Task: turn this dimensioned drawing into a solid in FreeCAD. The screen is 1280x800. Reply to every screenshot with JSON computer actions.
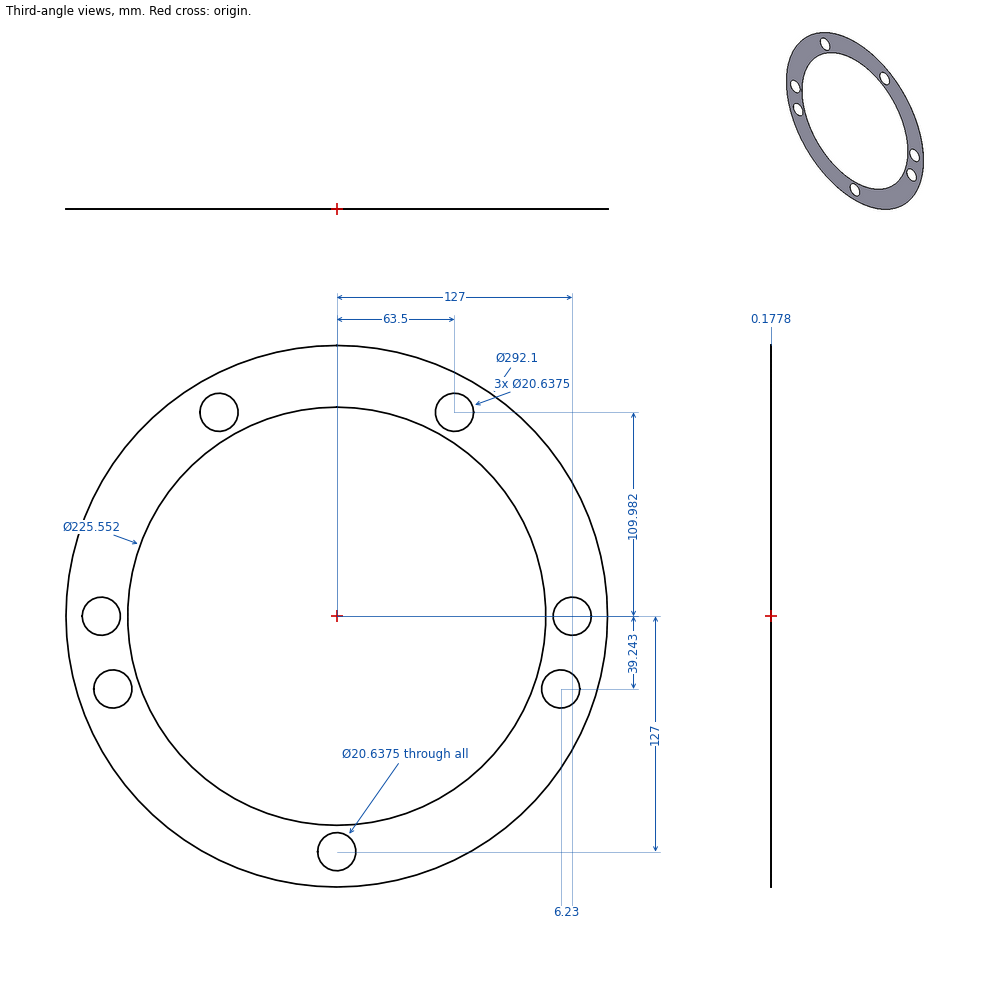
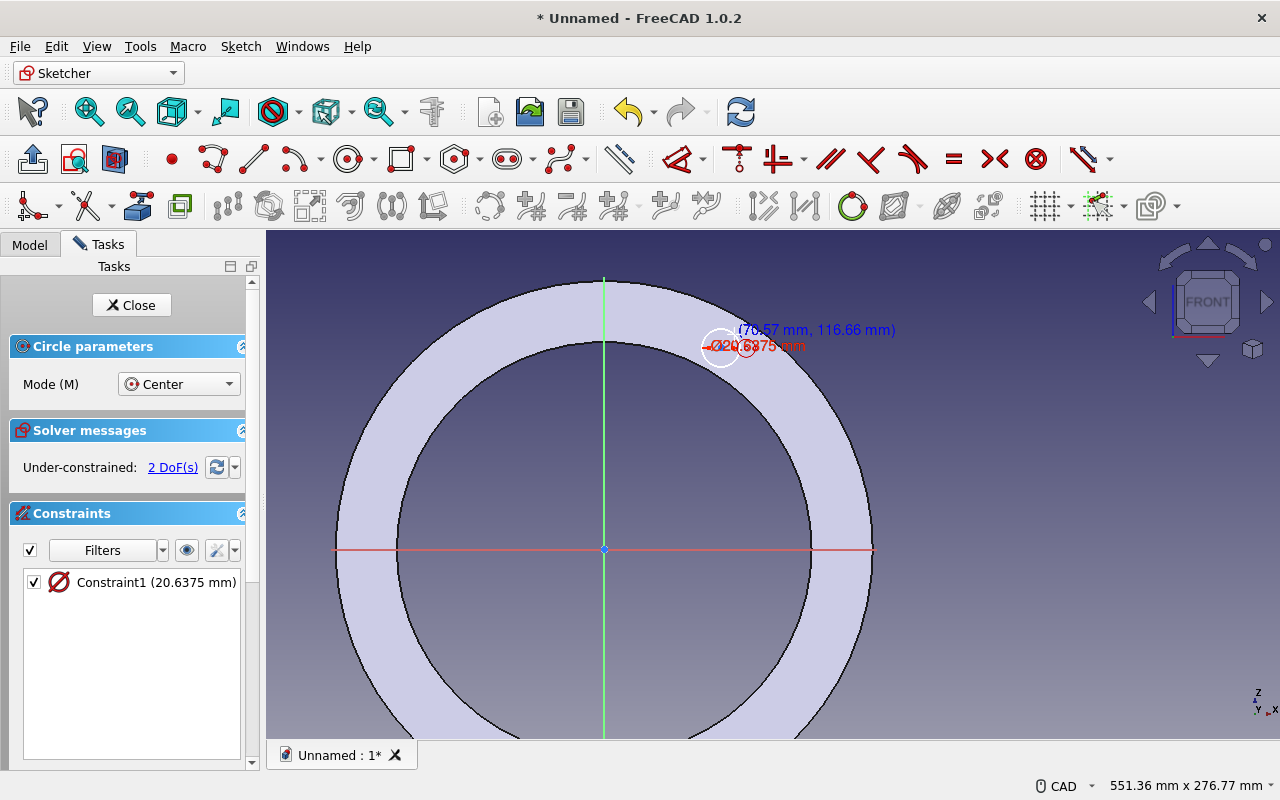
{"action": "left_click", "coordinate": [826, 622]}
{"action": "mouse_move", "coordinate": [840, 608]}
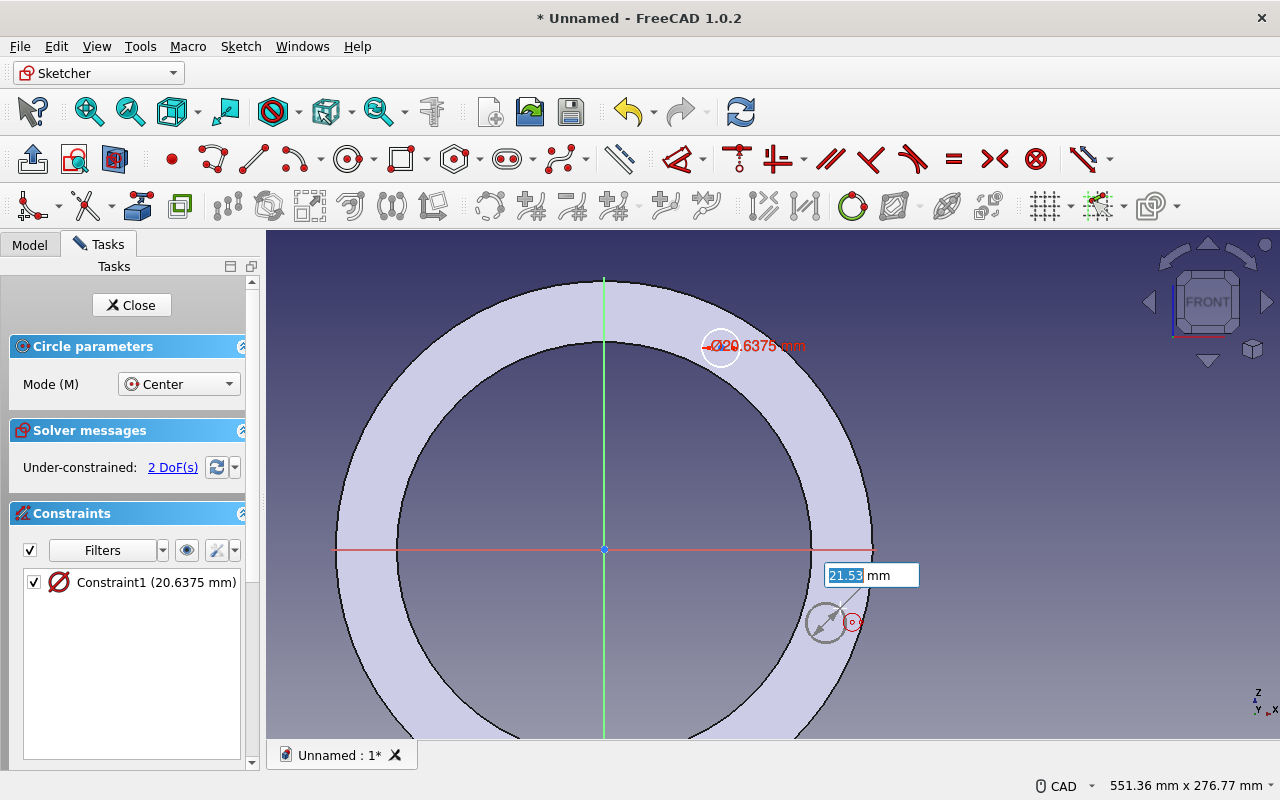
{"action": "type", "text": "20.6375"}
{"action": "key", "text": "Return"}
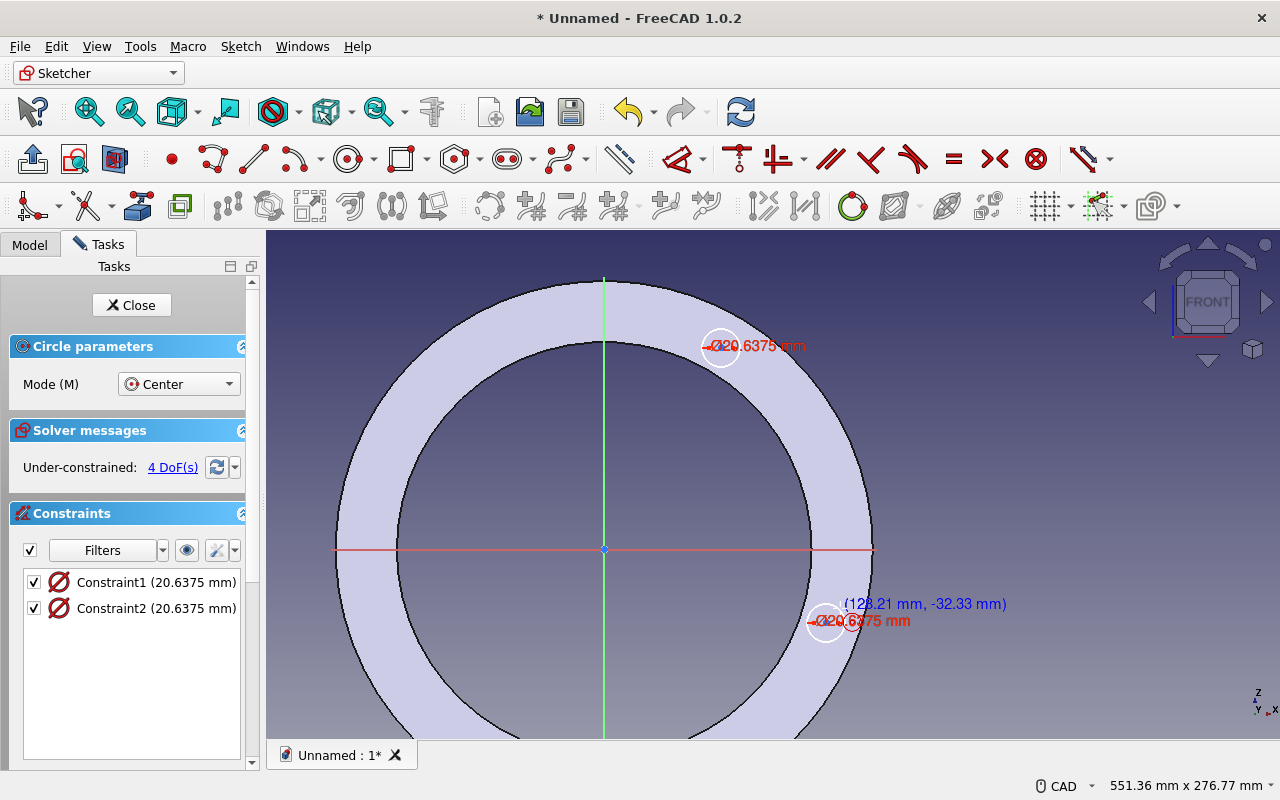
{"action": "left_click", "coordinate": [838, 550]}
{"action": "mouse_move", "coordinate": [844, 532]}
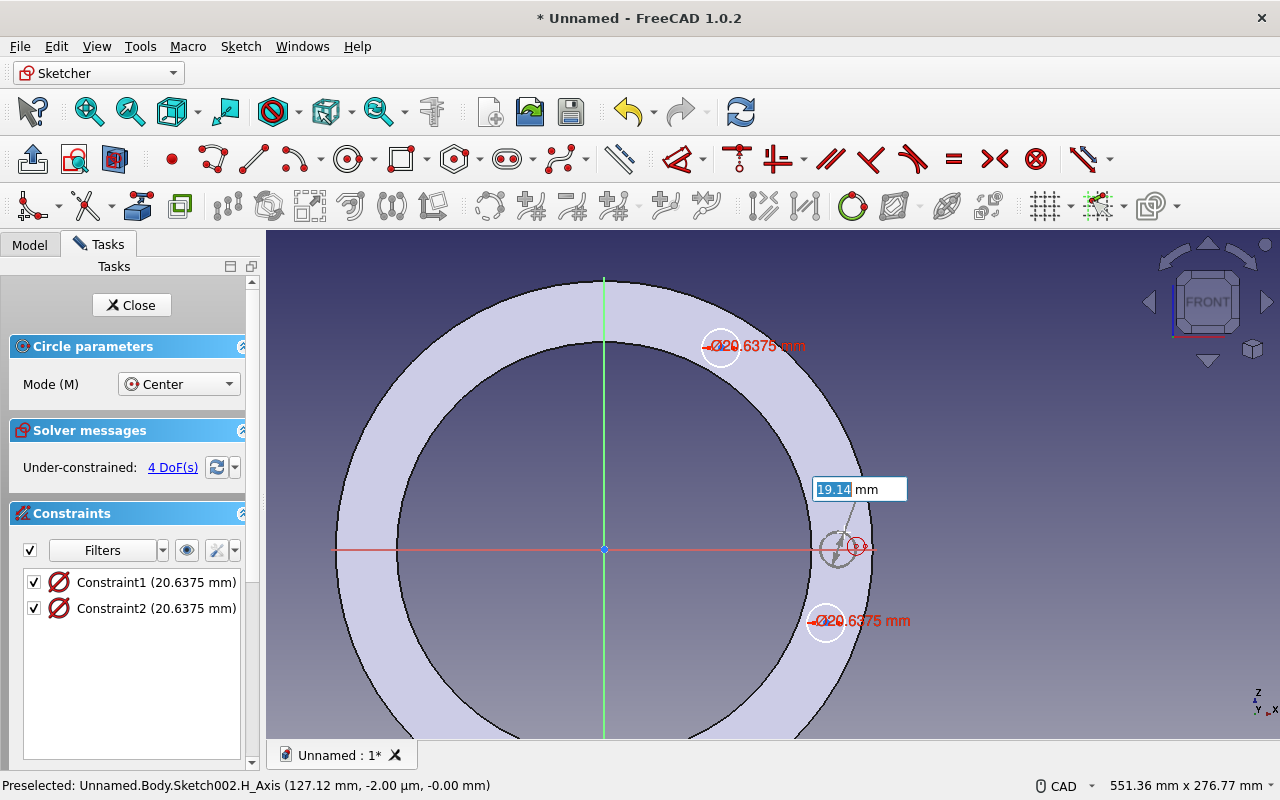
{"action": "type", "text": "20.6375"}
{"action": "key", "text": "Return"}
{"action": "key", "text": "Escape"}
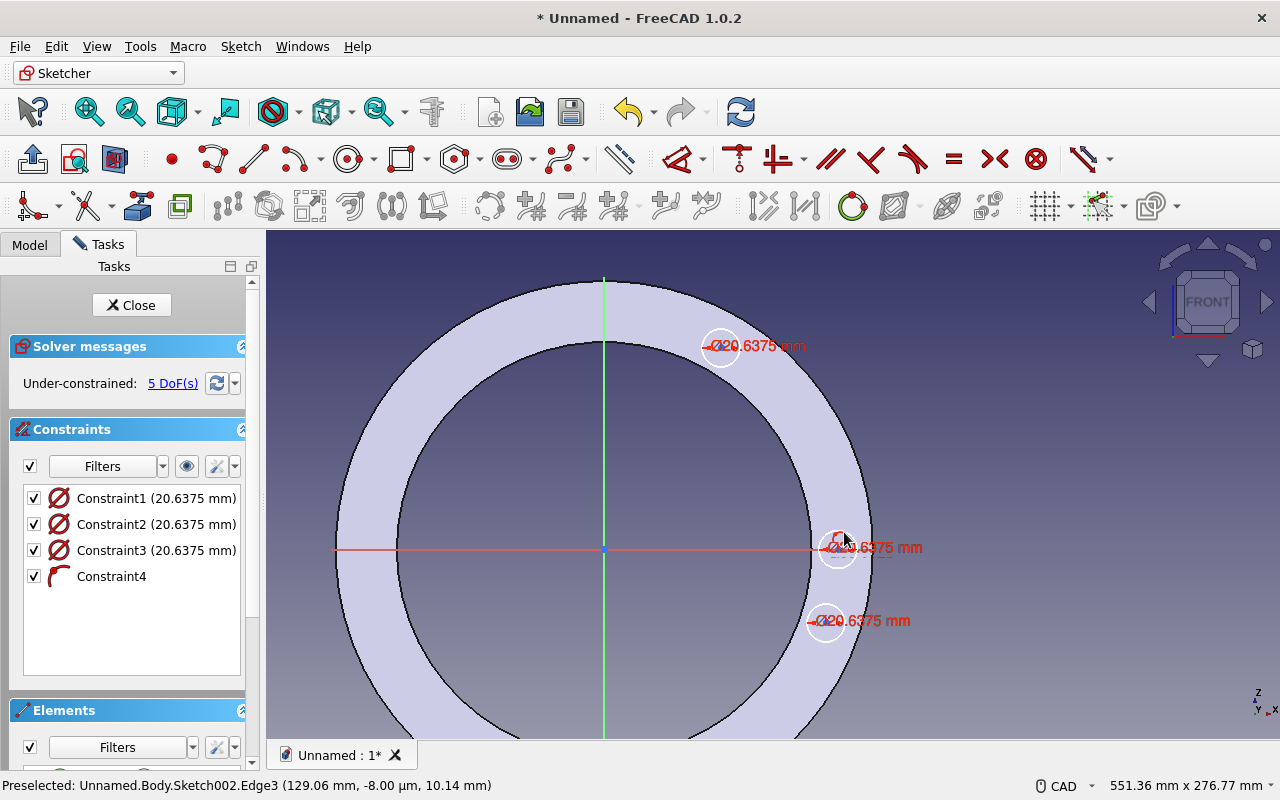
{"action": "left_click", "coordinate": [676, 160]}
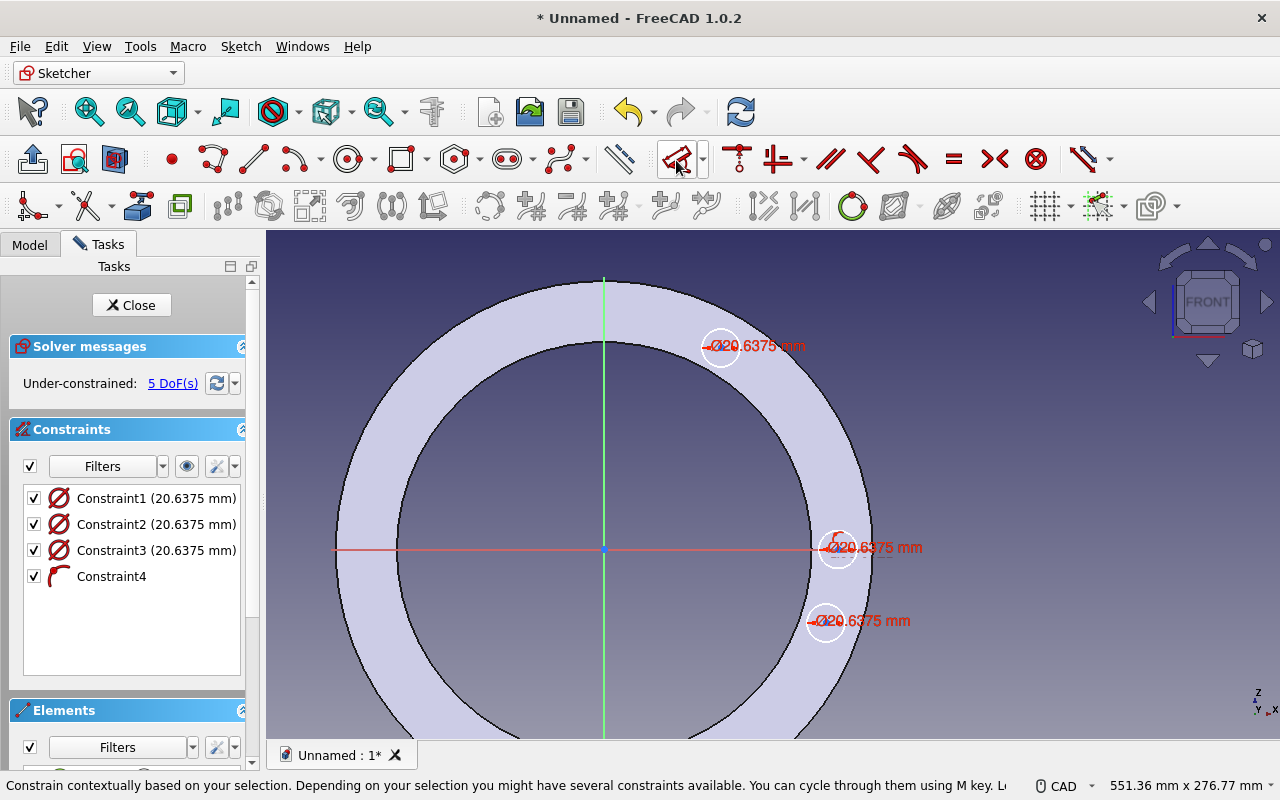
{"action": "left_click", "coordinate": [838, 550]}
{"action": "left_click", "coordinate": [721, 584]}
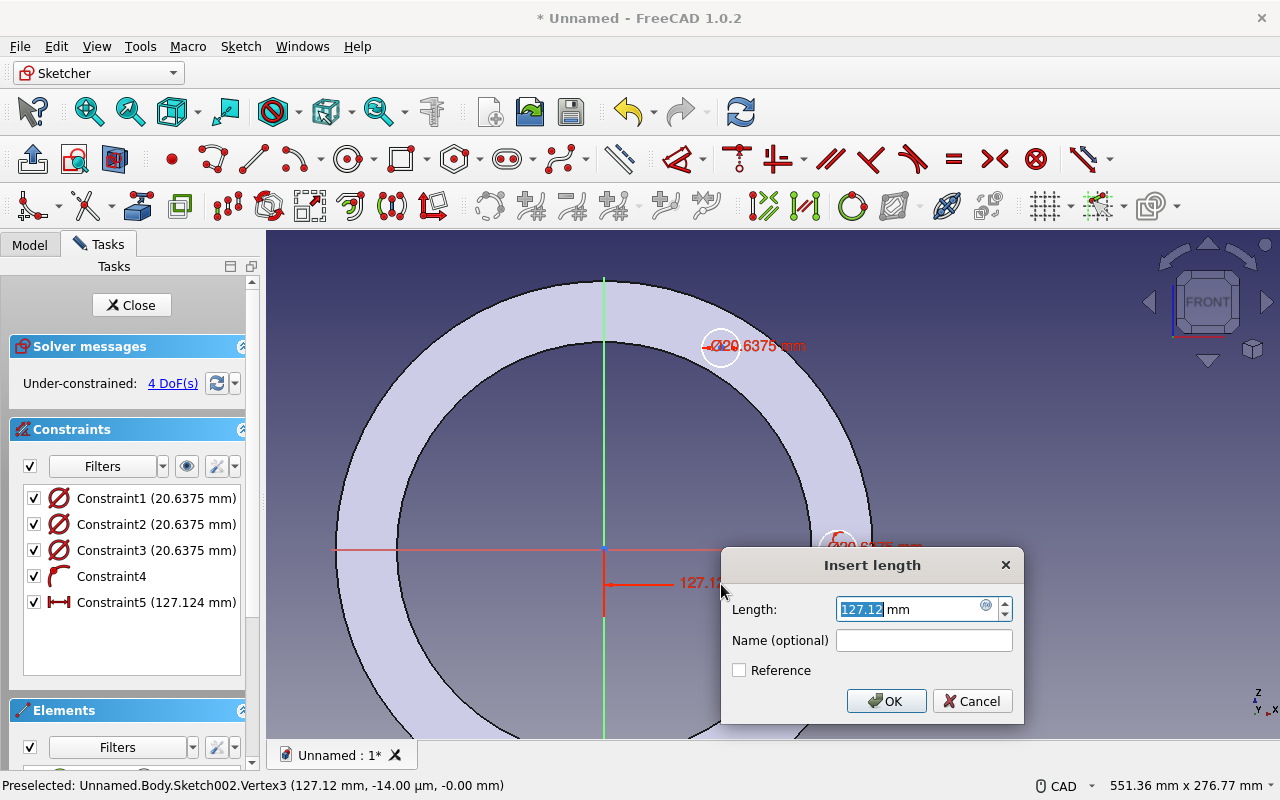
{"action": "type", "text": "127"}
{"action": "key", "text": "Return"}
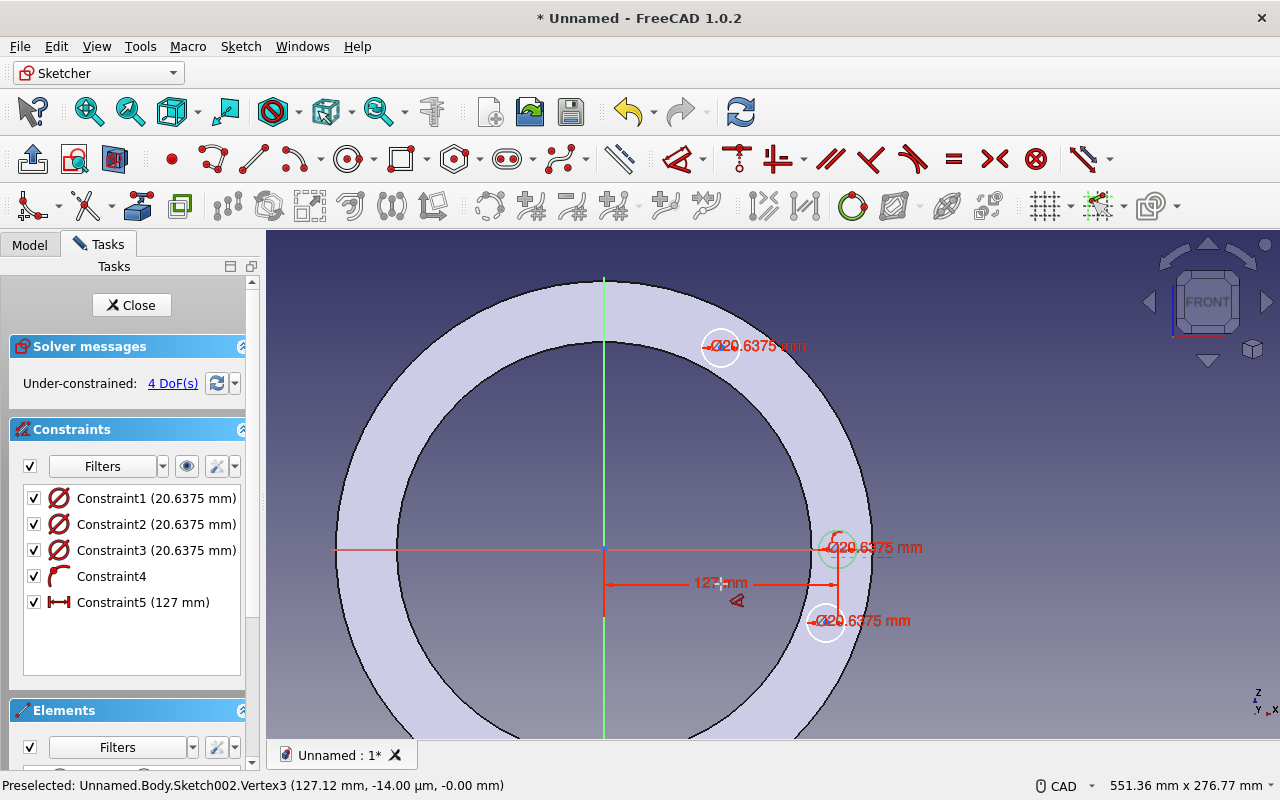
{"action": "left_click", "coordinate": [721, 348]}
{"action": "left_click", "coordinate": [663, 314]}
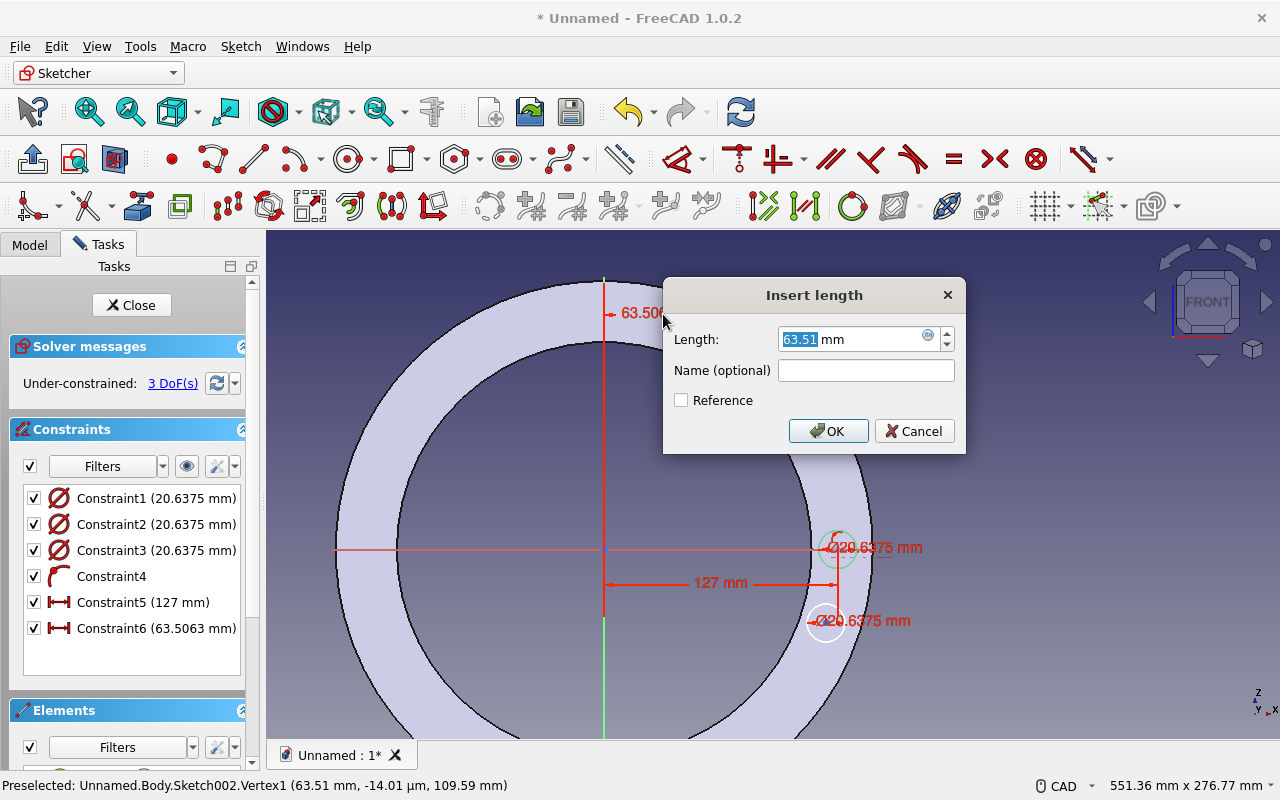
{"action": "type", "text": "63.5"}
{"action": "key", "text": "Return"}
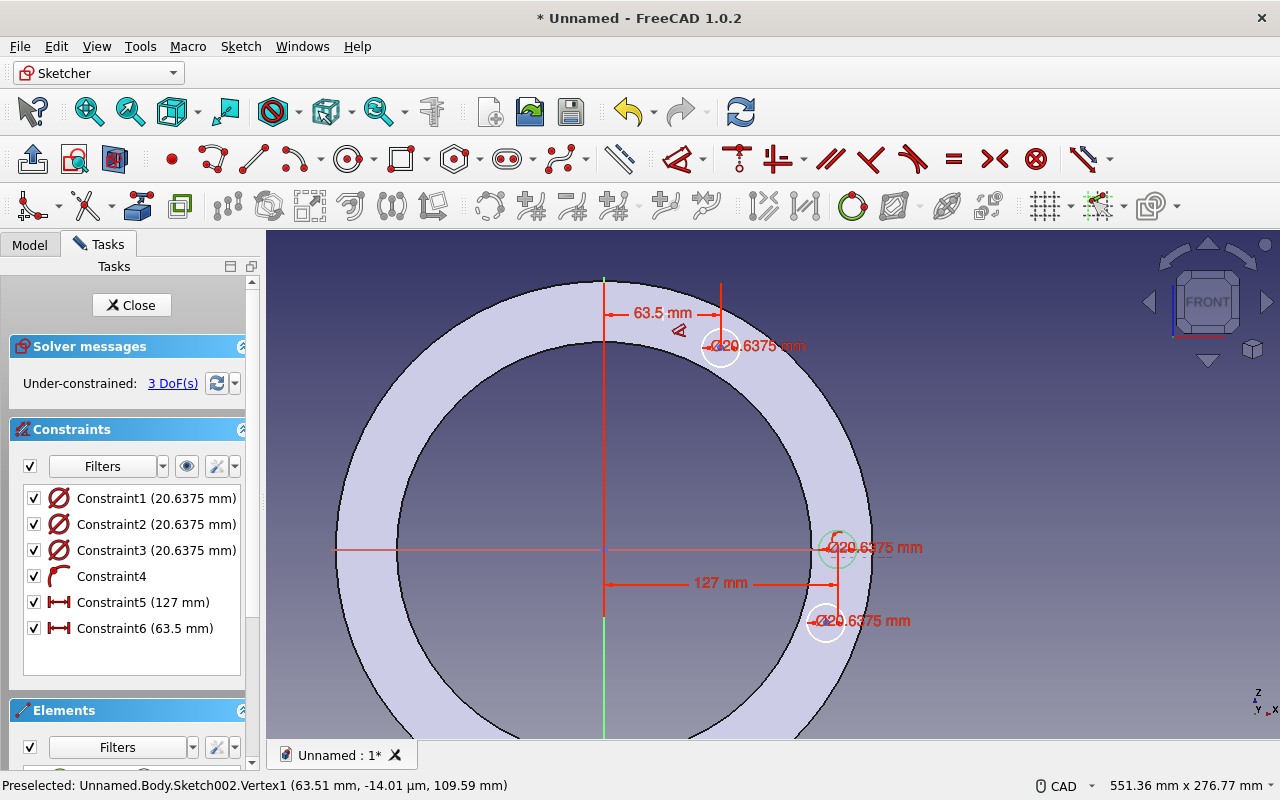
{"action": "scroll", "coordinate": [826, 623], "scroll_direction": "up", "scroll_amount": 7}